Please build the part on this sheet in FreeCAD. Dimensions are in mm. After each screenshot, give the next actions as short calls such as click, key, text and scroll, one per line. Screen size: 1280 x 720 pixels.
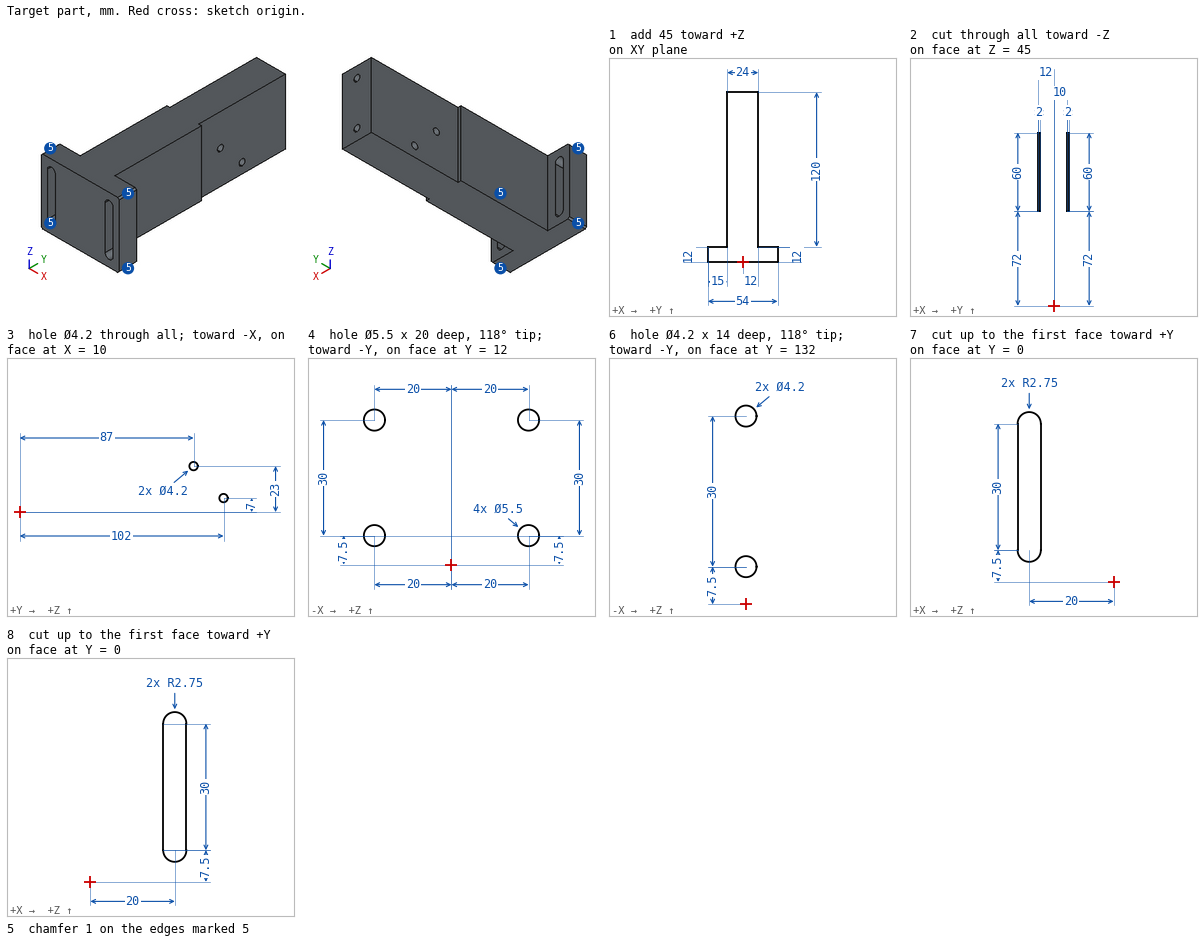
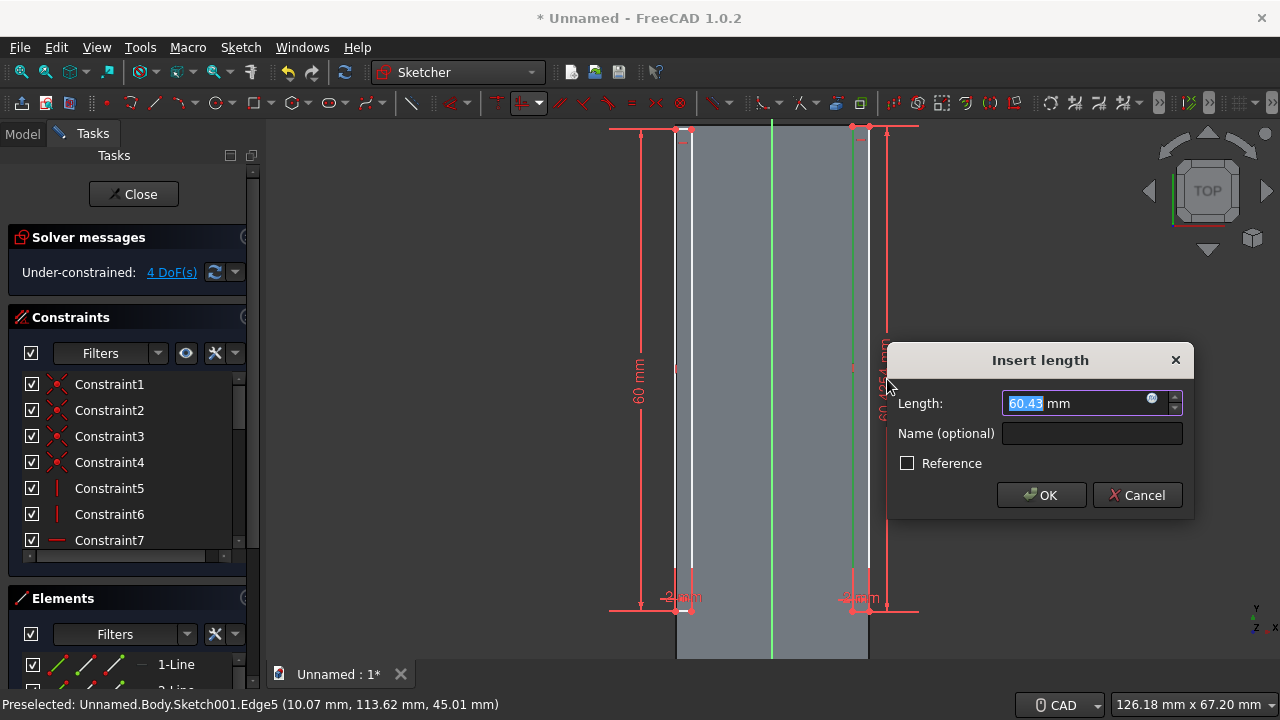
text(60)
key(Return)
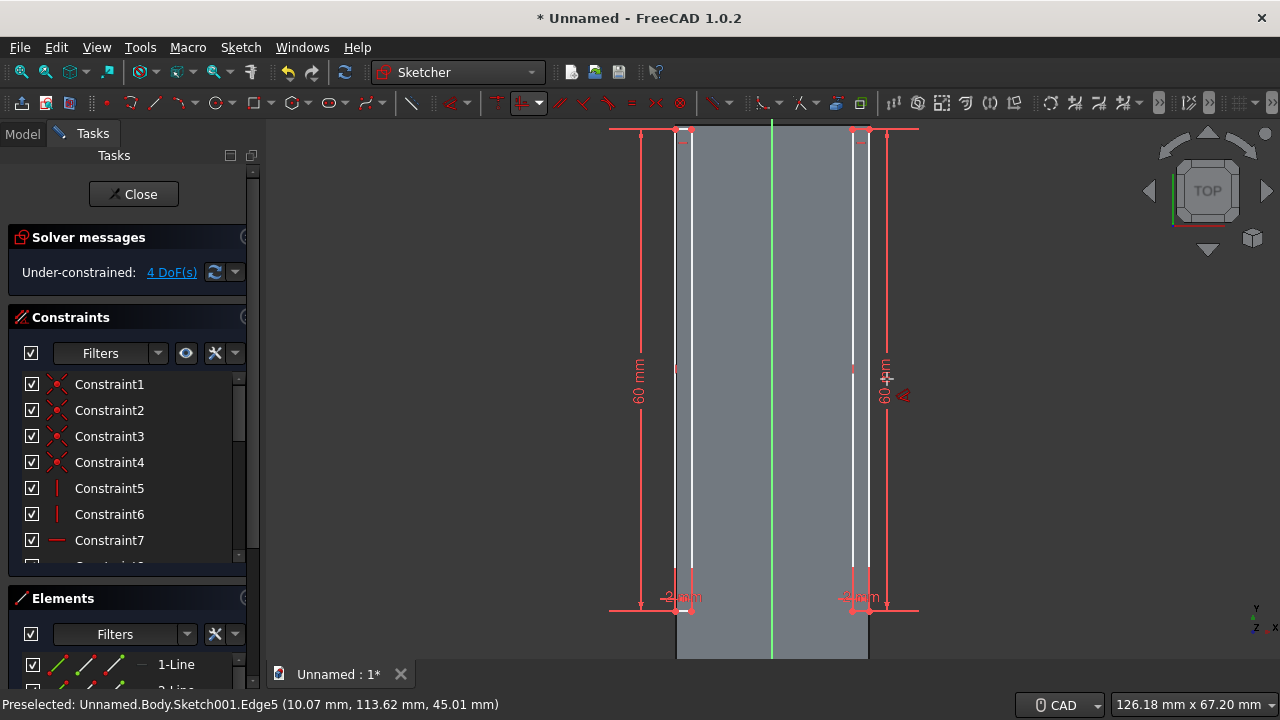
scroll(675, 274, down, 6)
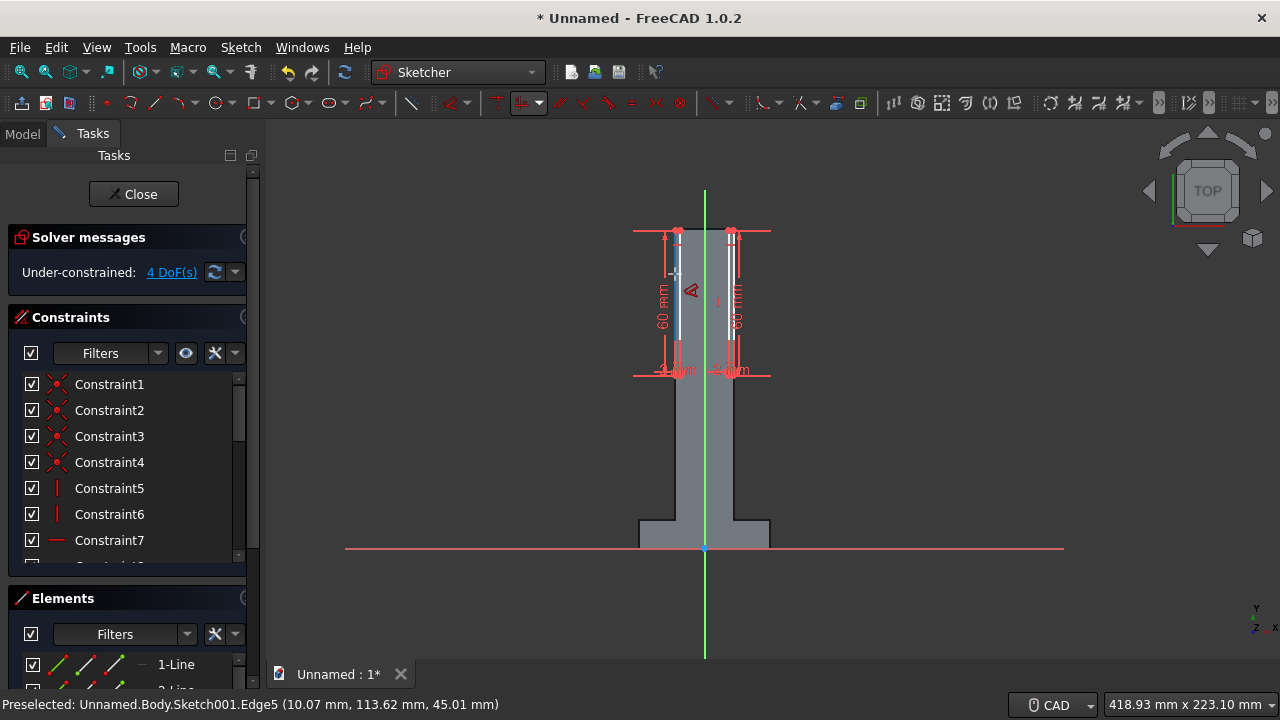
scroll(675, 231, up, 5)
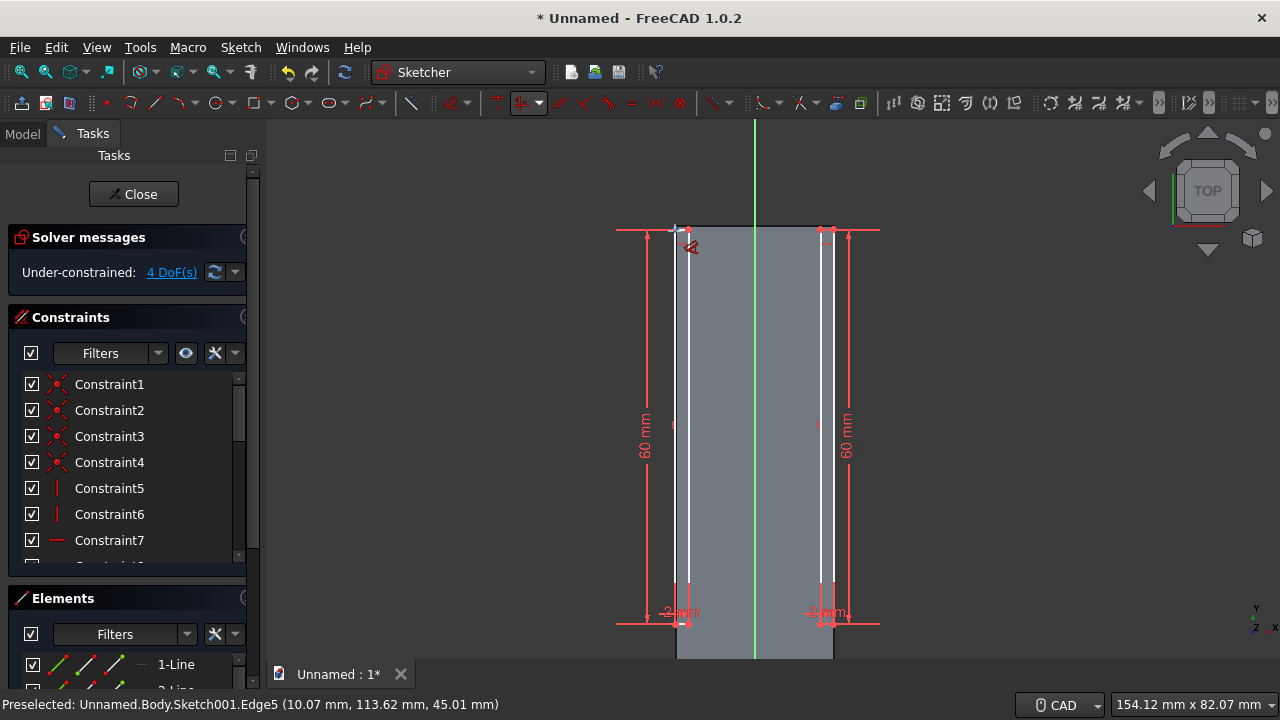
click(675, 230)
click(715, 196)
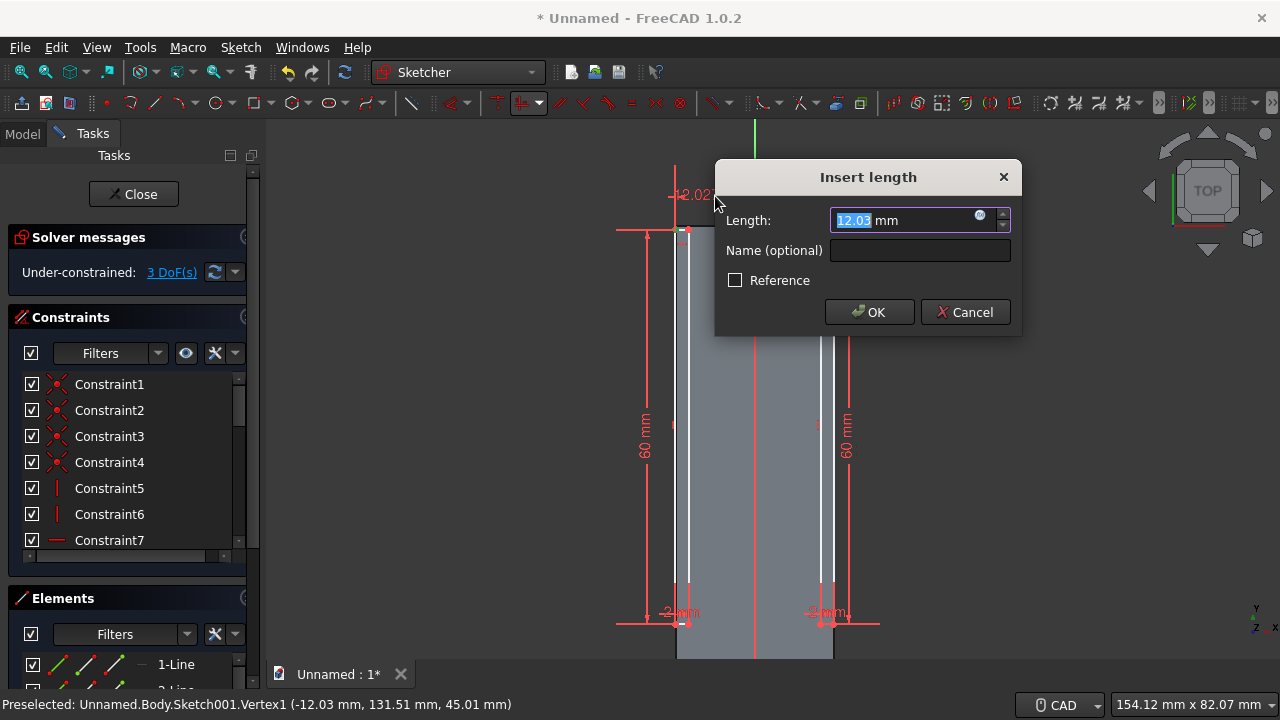
text(12)
key(Return)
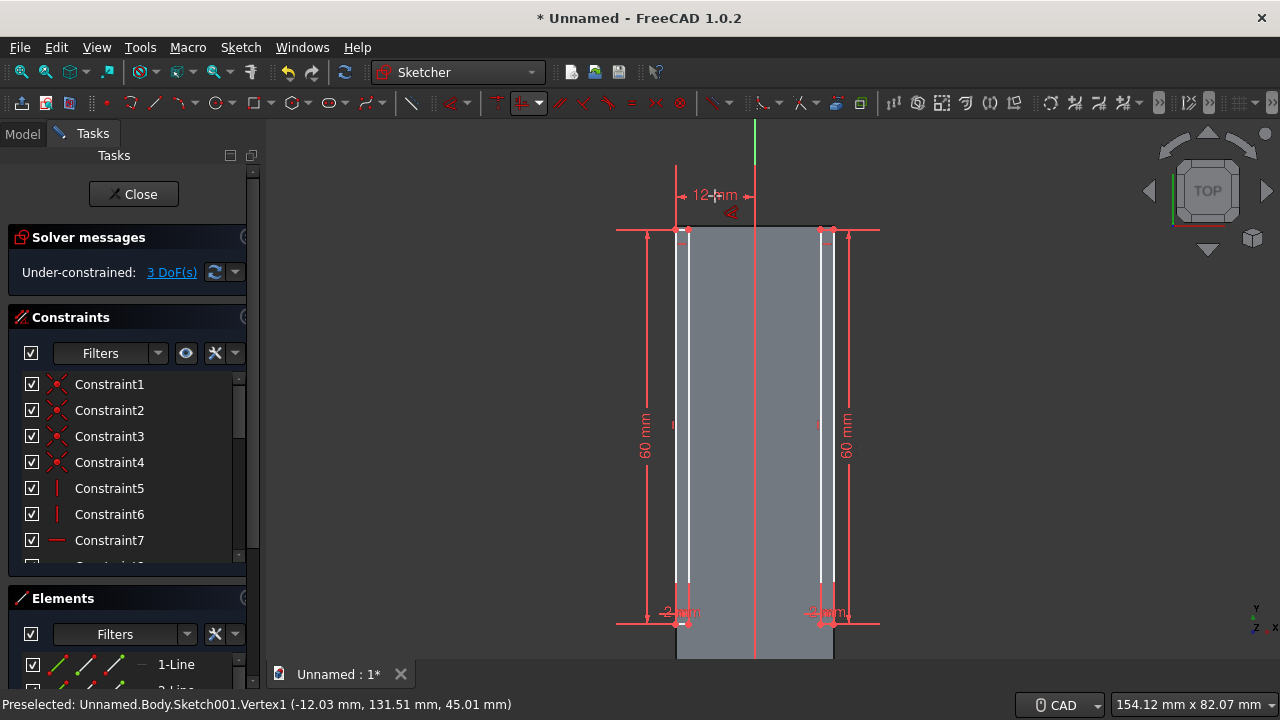
click(676, 624)
click(594, 628)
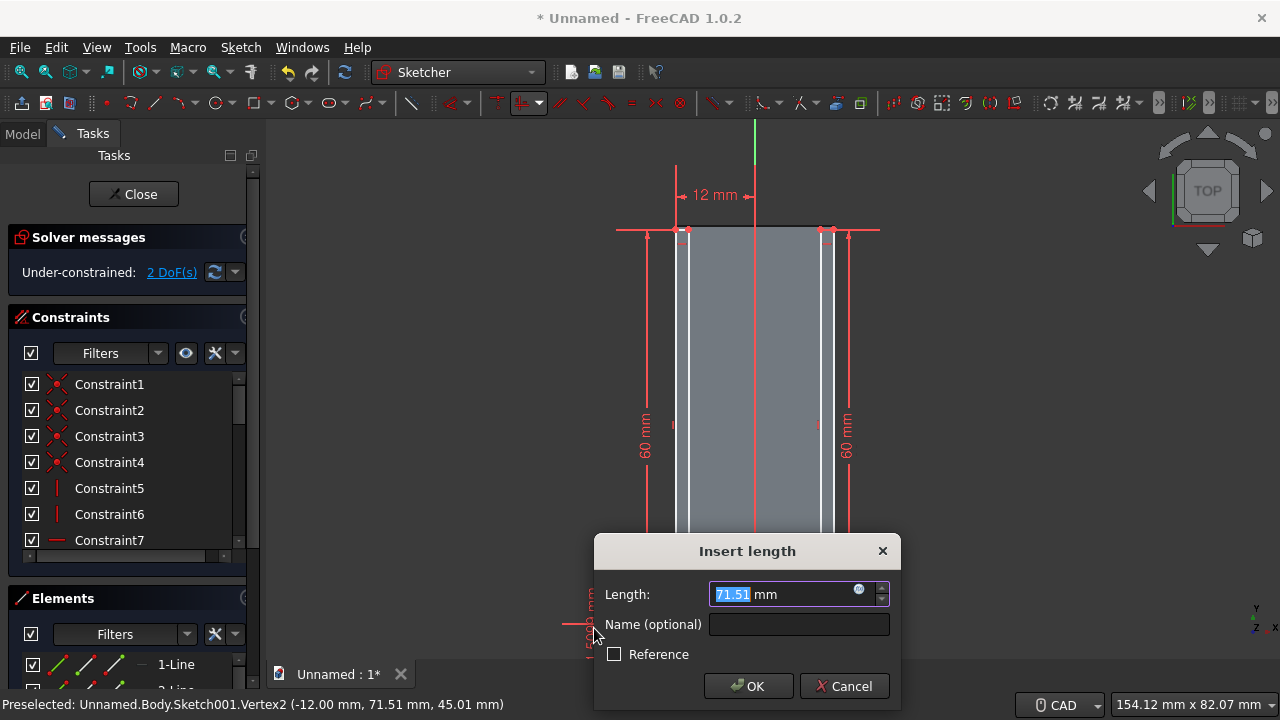
text(72)
key(Return)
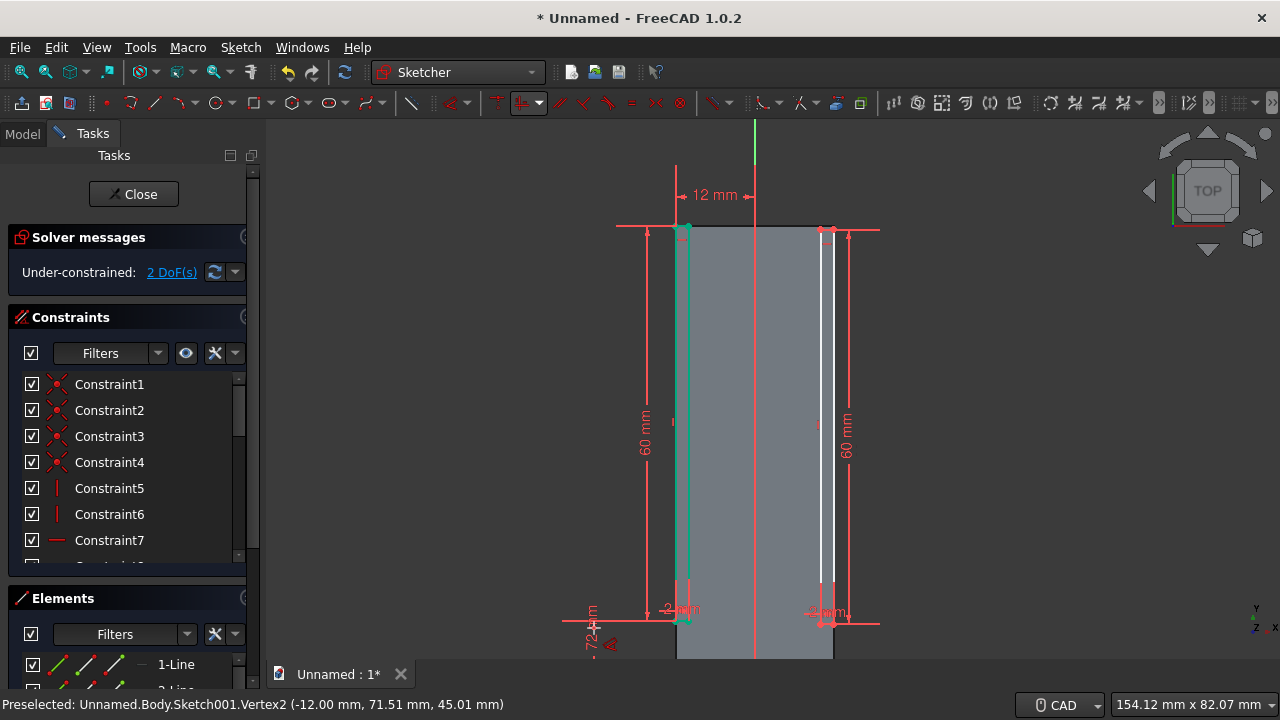
click(821, 230)
click(788, 196)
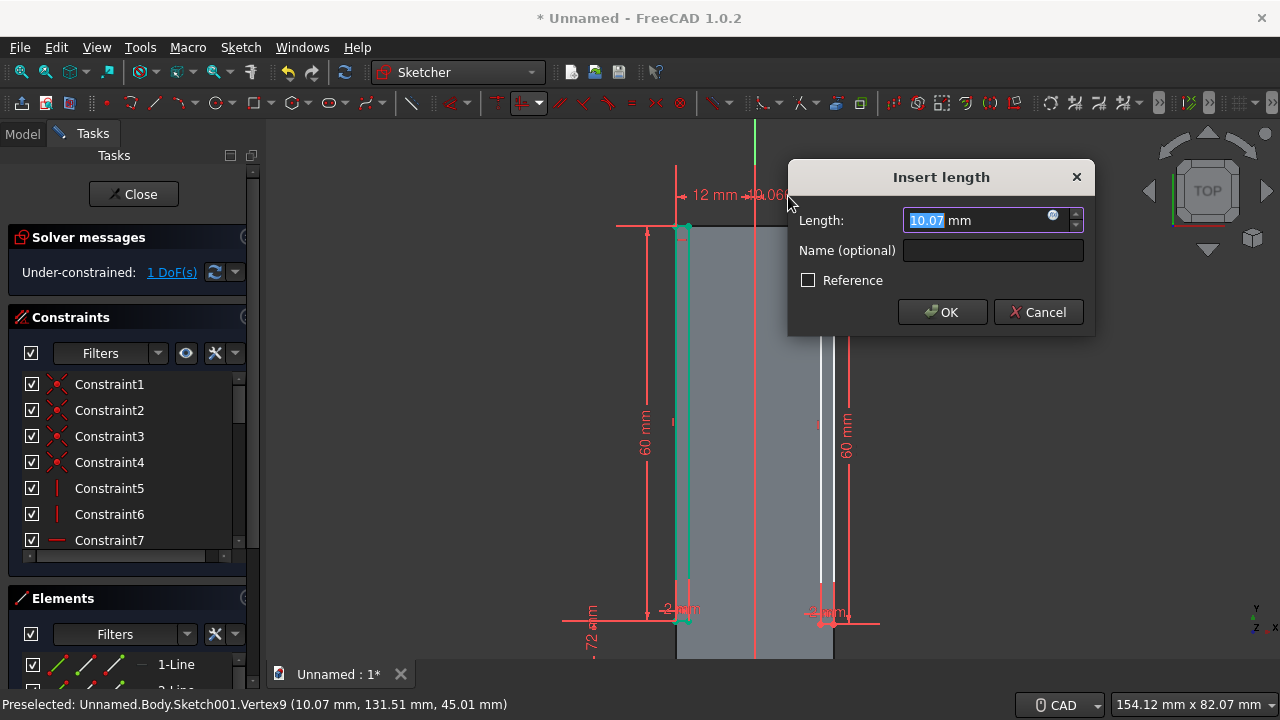
text(10)
key(Return)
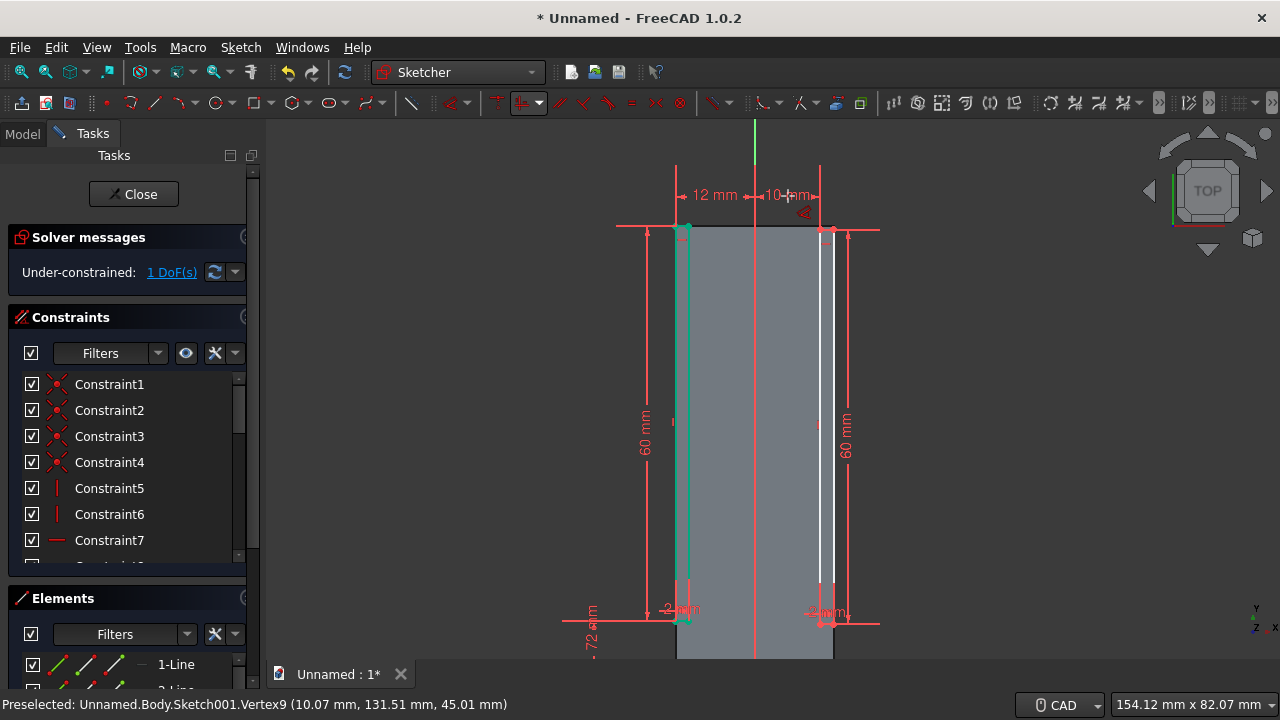
click(820, 624)
click(902, 628)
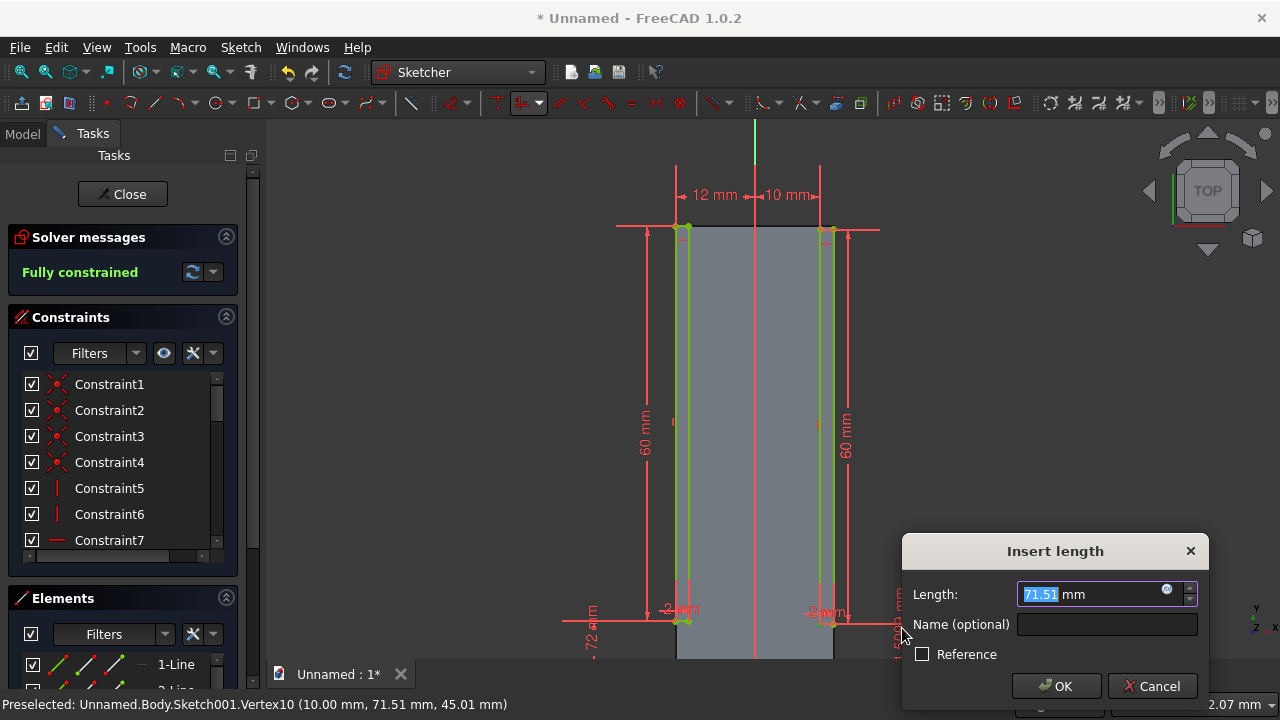
text(72)
key(Return)
key(Escape)